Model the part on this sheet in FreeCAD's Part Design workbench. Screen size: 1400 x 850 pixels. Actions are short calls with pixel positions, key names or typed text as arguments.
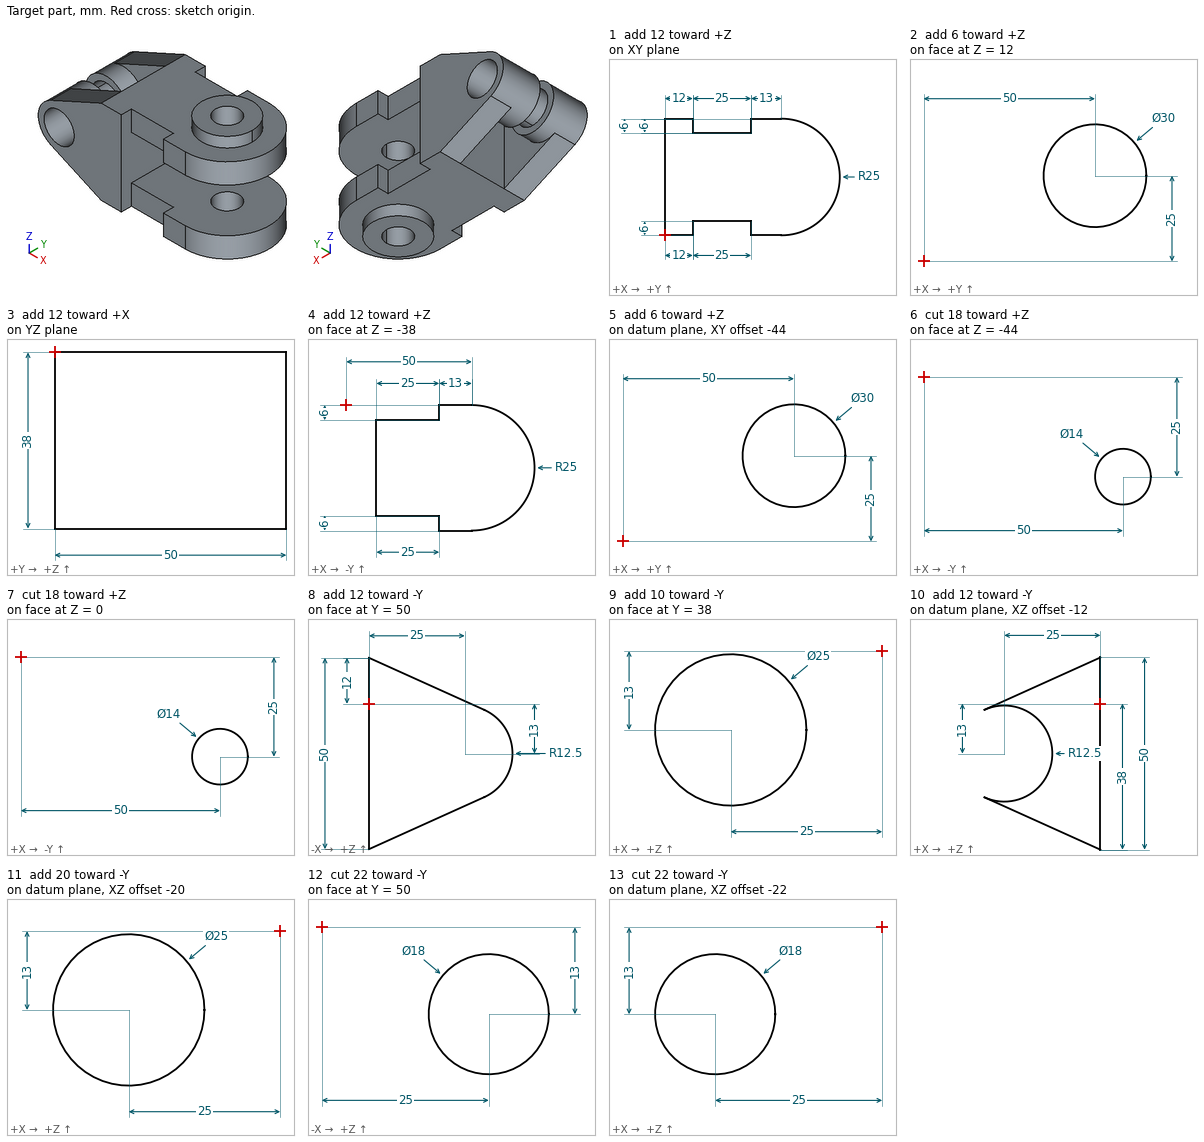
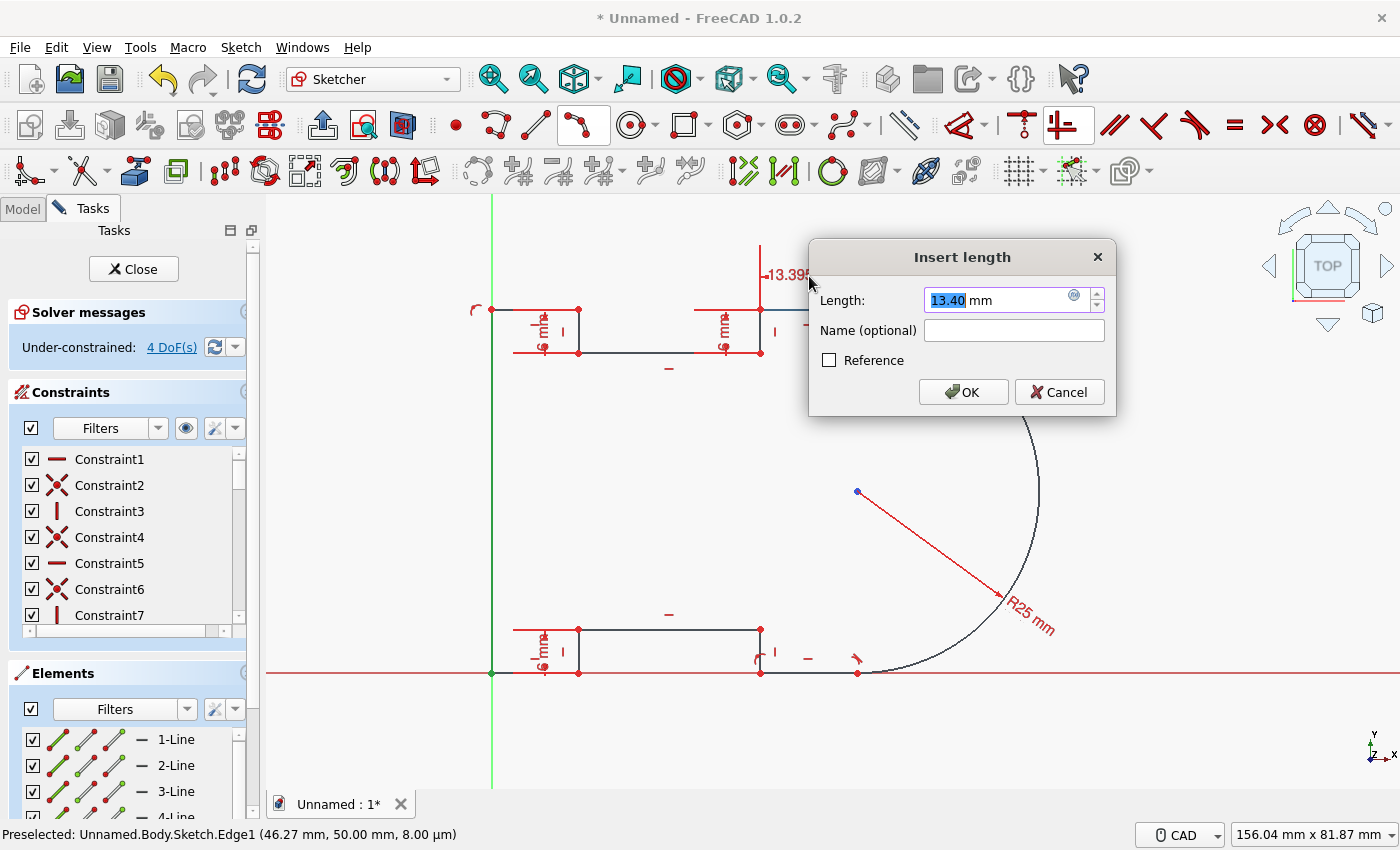
text(13)
key(Return)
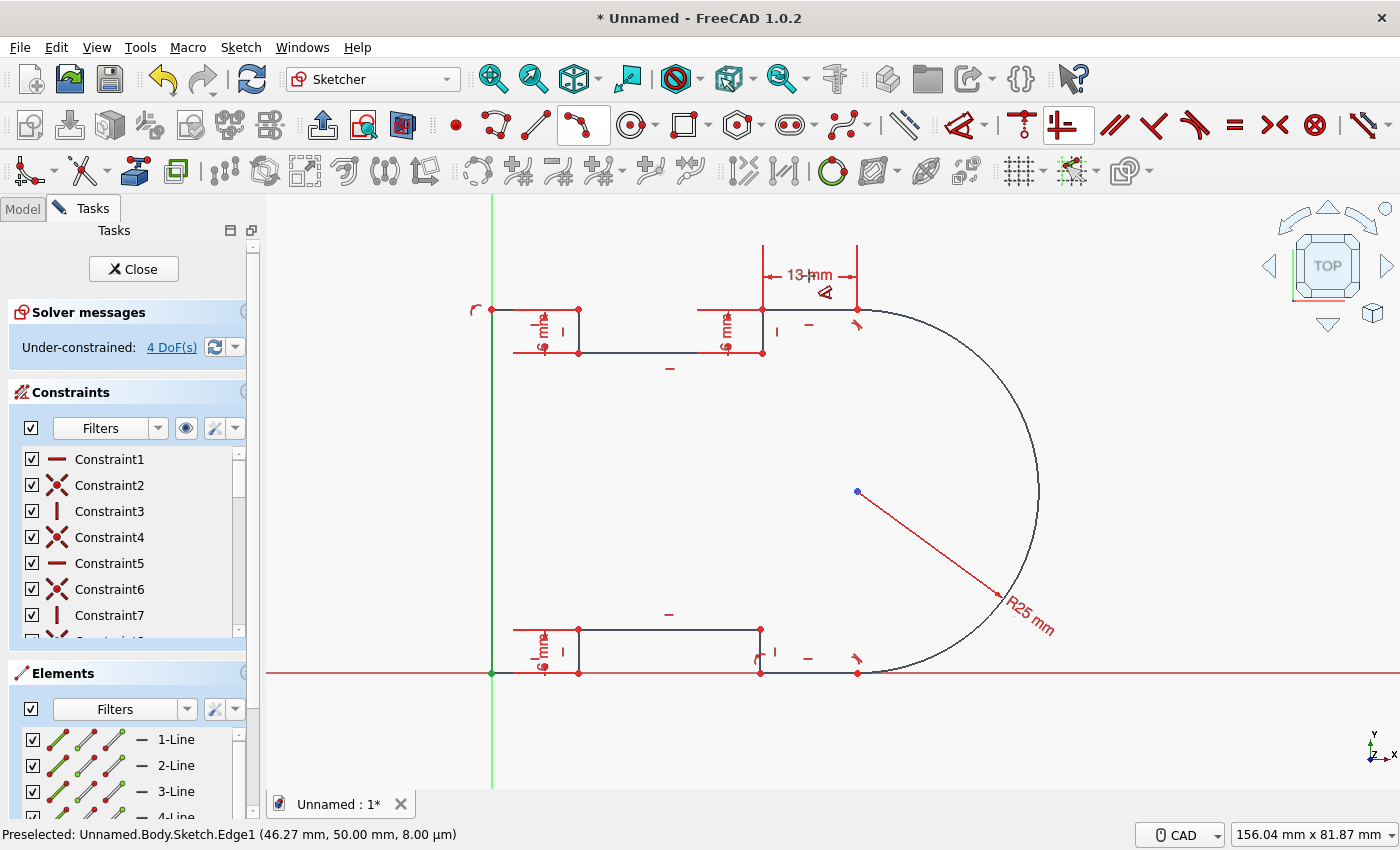
click(707, 353)
click(628, 319)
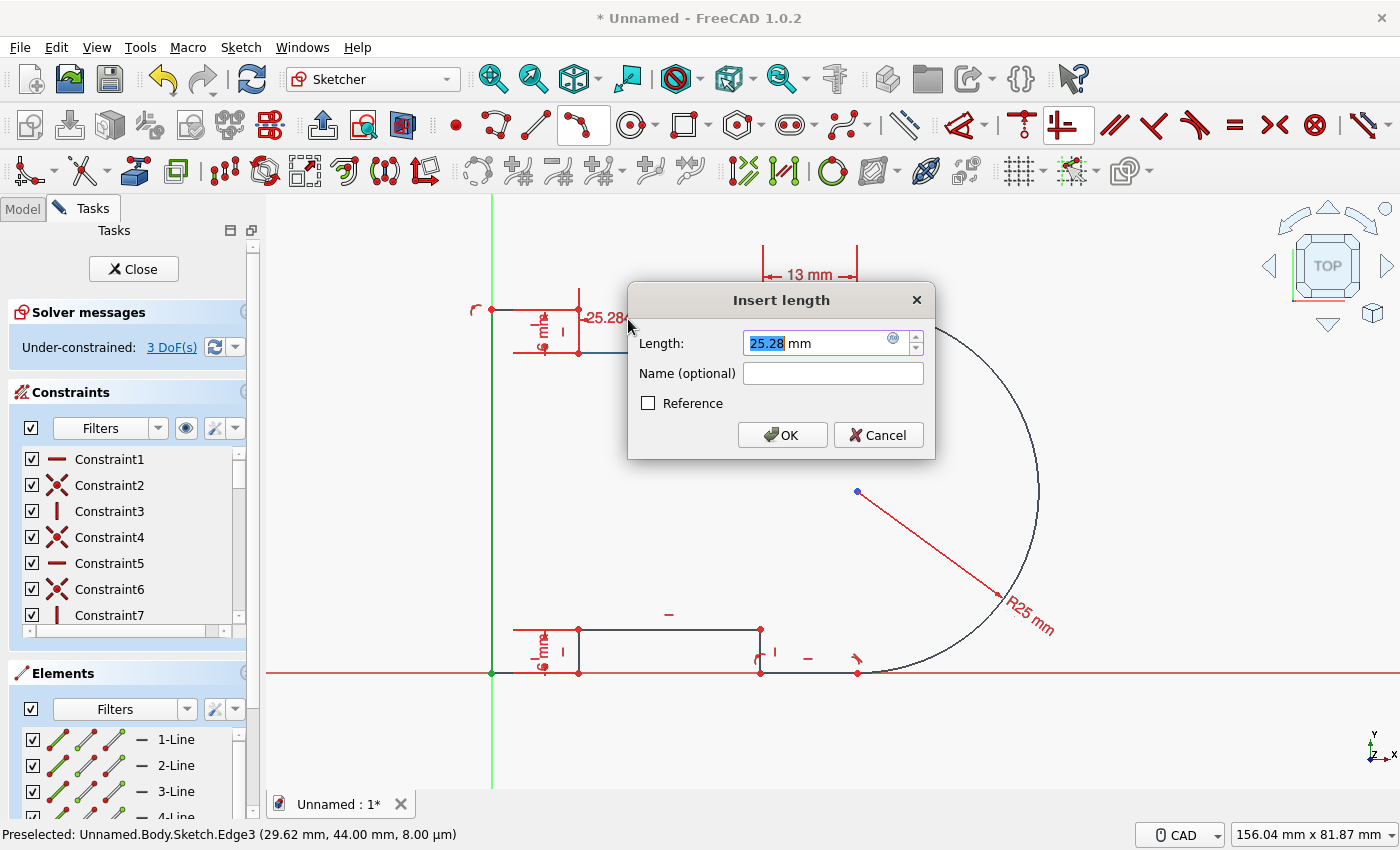
text(25)
key(Return)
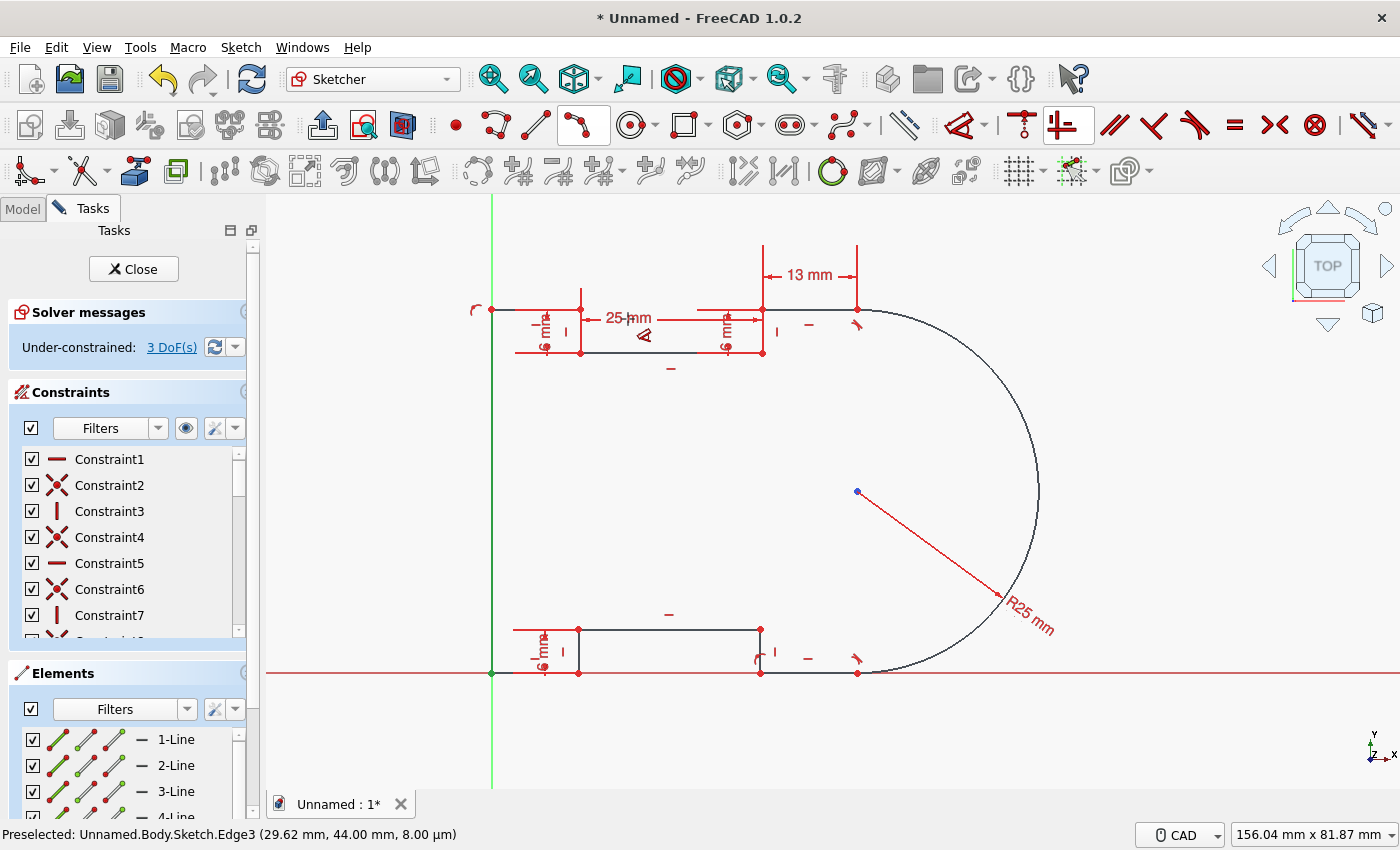
click(554, 310)
click(536, 276)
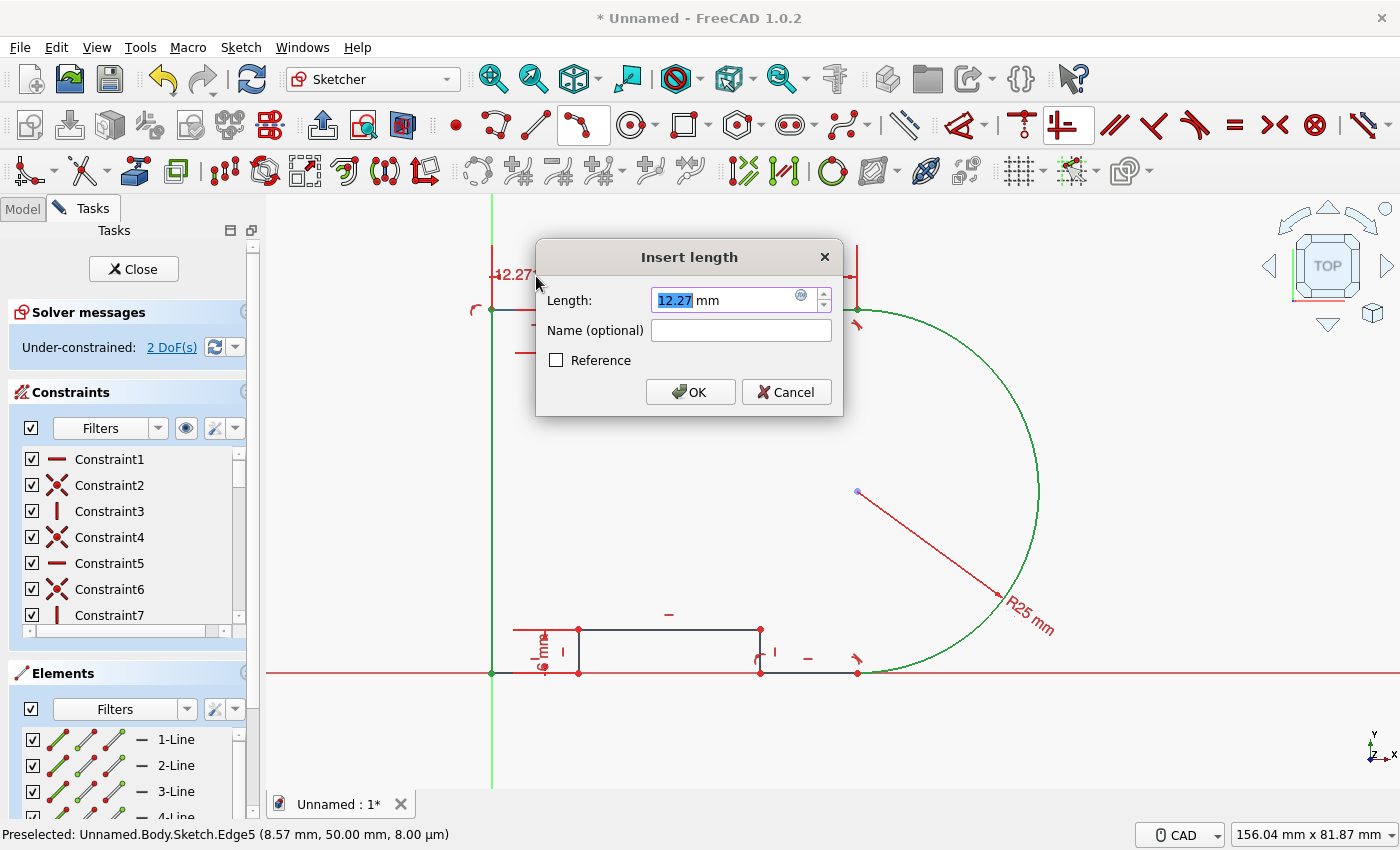
text(12)
key(Return)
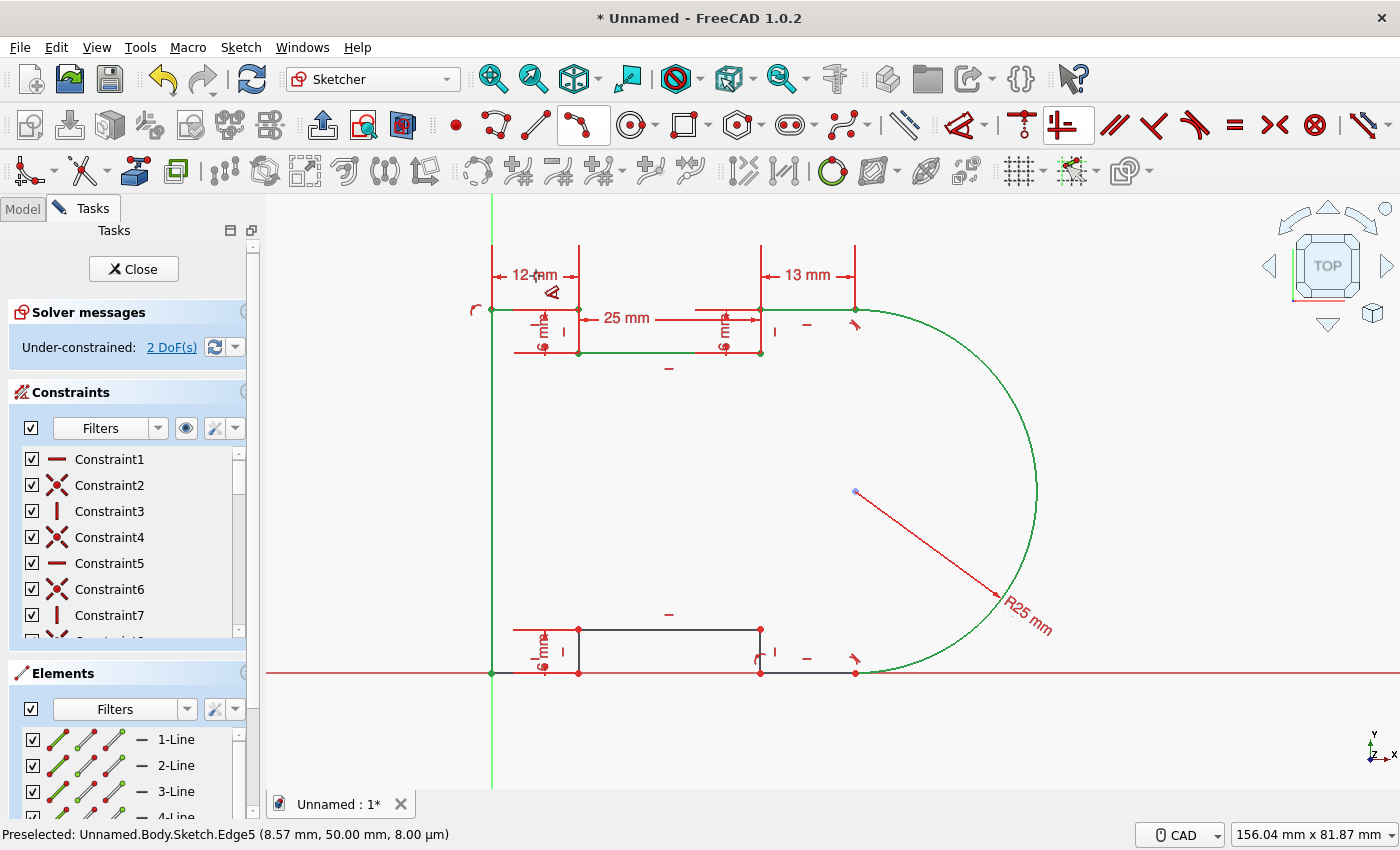
click(518, 673)
click(535, 707)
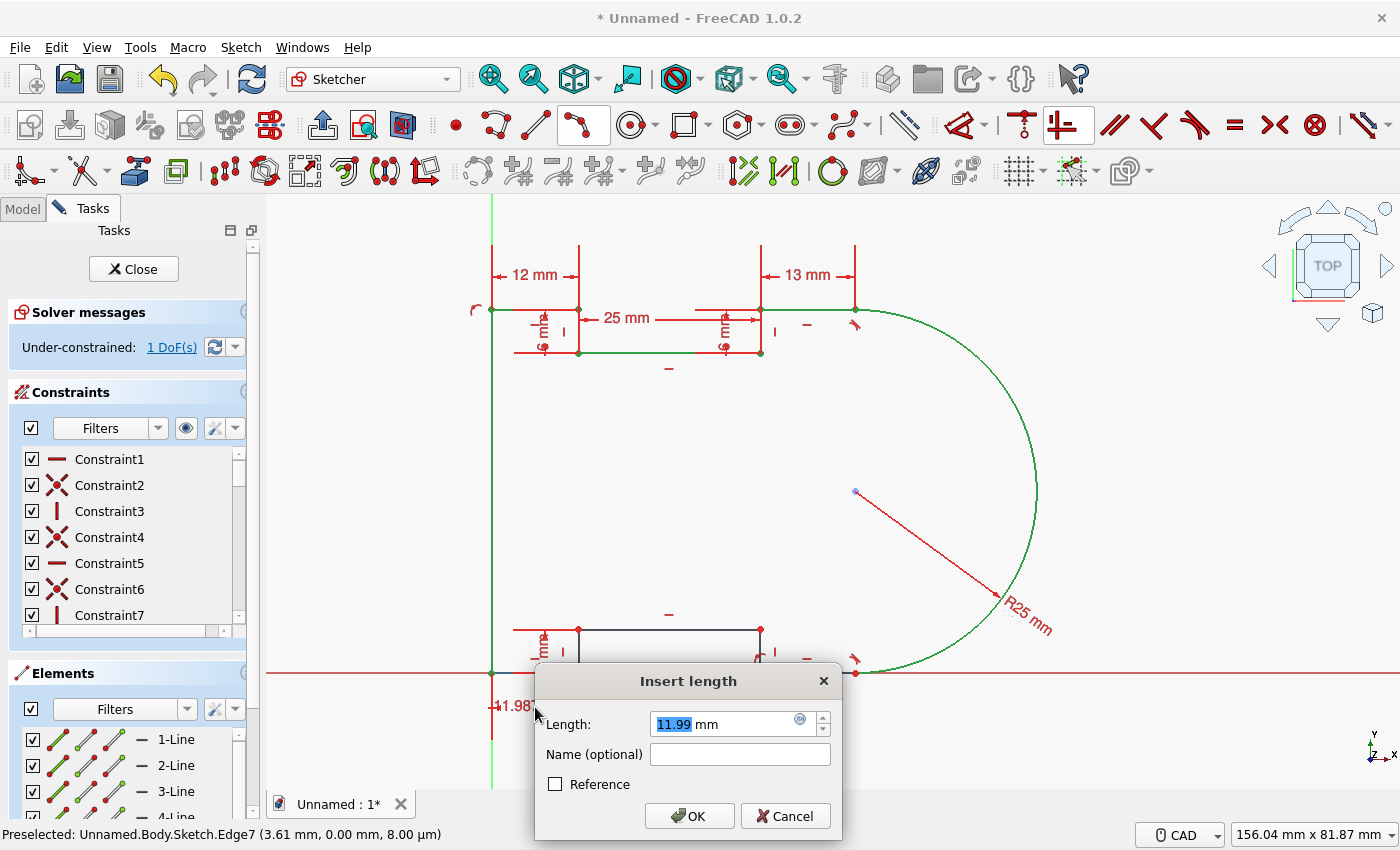
text(12)
key(Return)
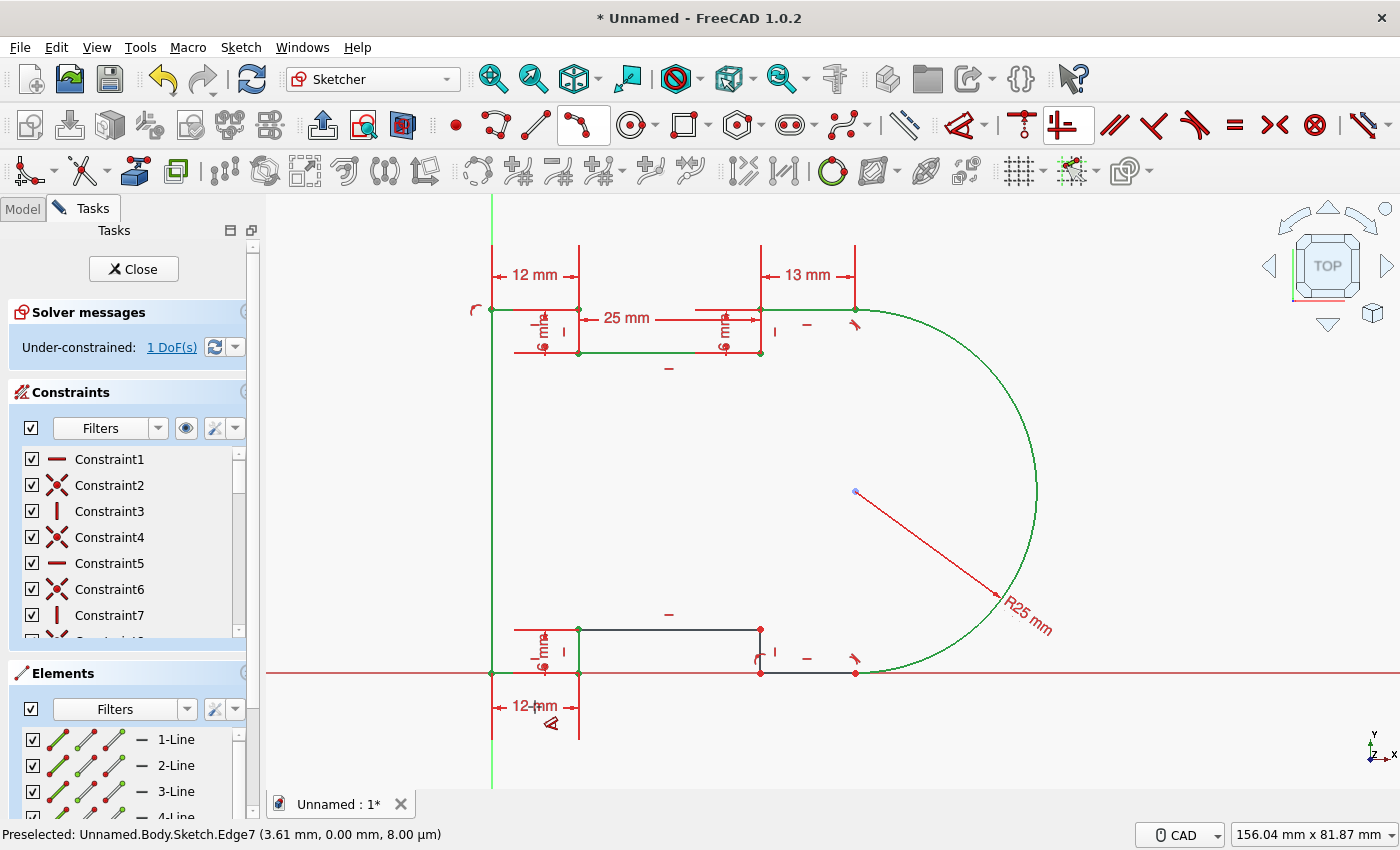
click(633, 630)
click(670, 596)